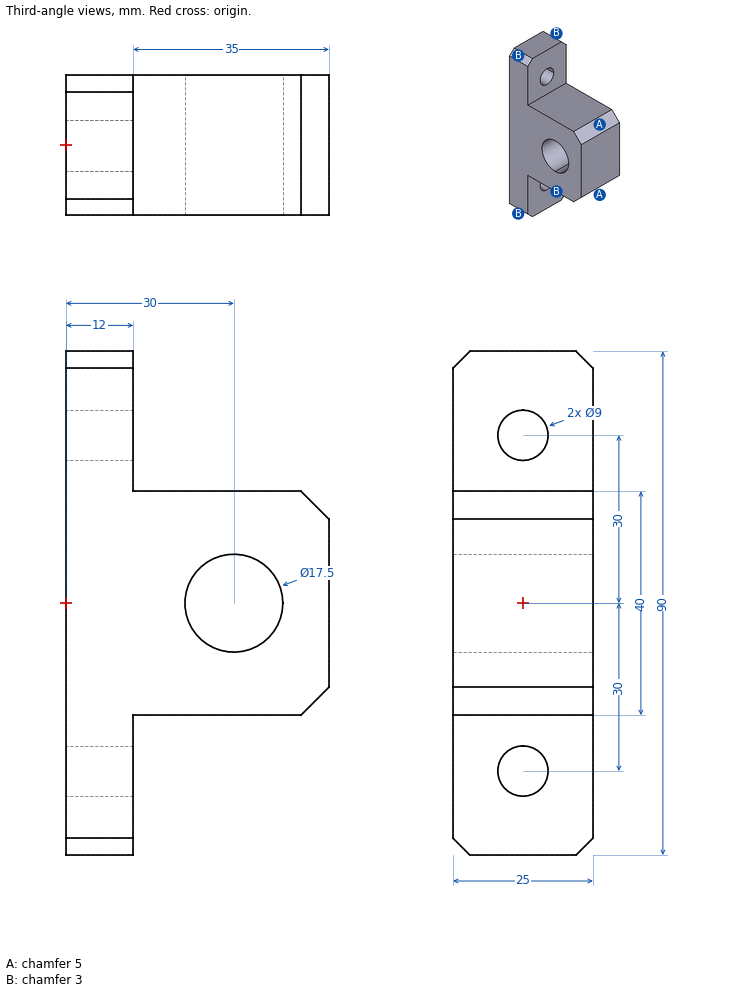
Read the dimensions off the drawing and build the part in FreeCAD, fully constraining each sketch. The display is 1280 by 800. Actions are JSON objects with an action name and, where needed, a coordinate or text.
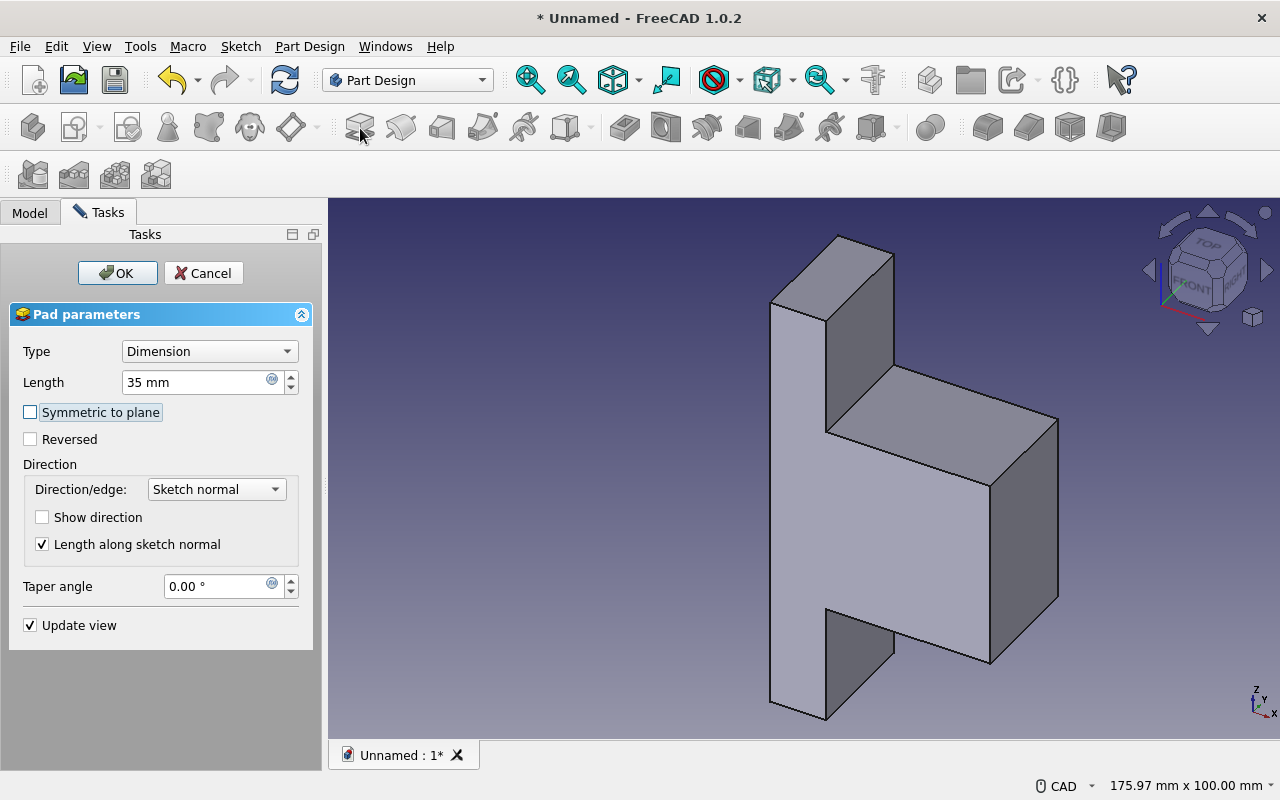
{"action": "left_click", "coordinate": [118, 273]}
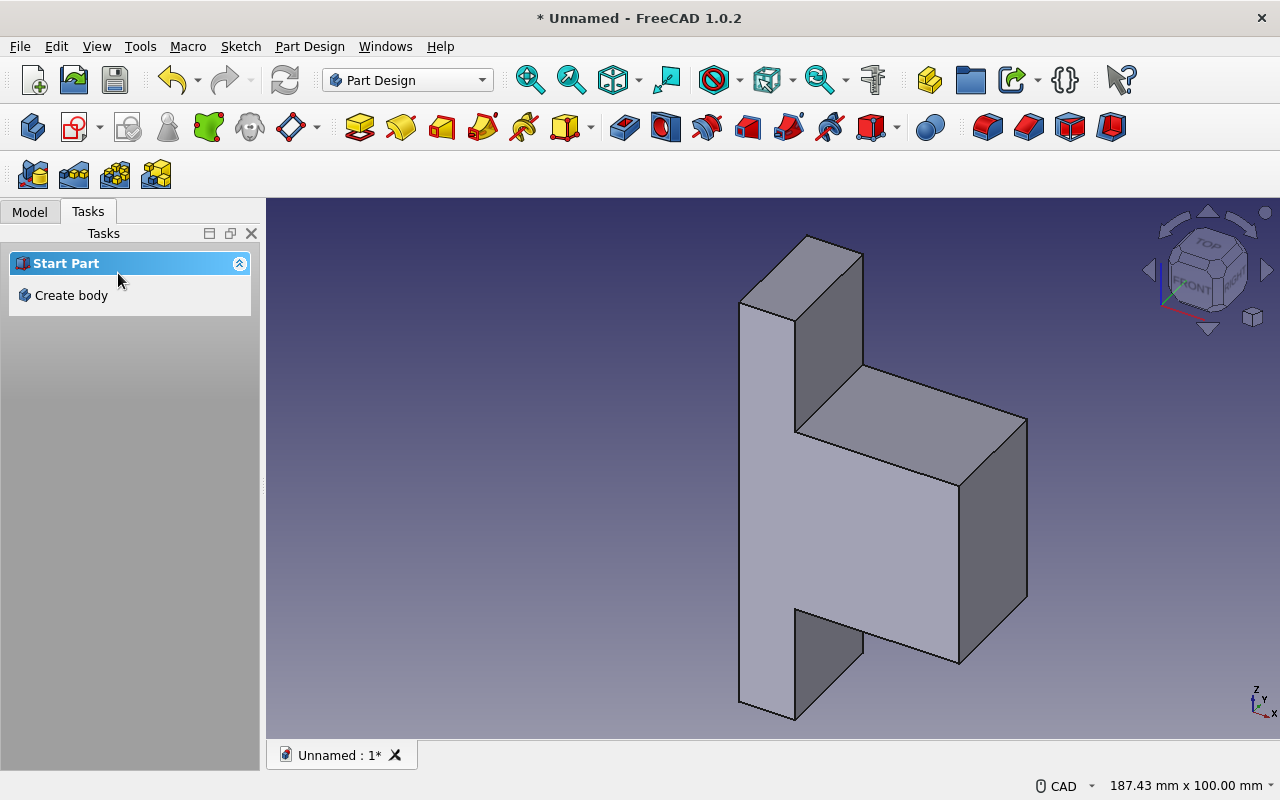
{"action": "left_click", "coordinate": [531, 80]}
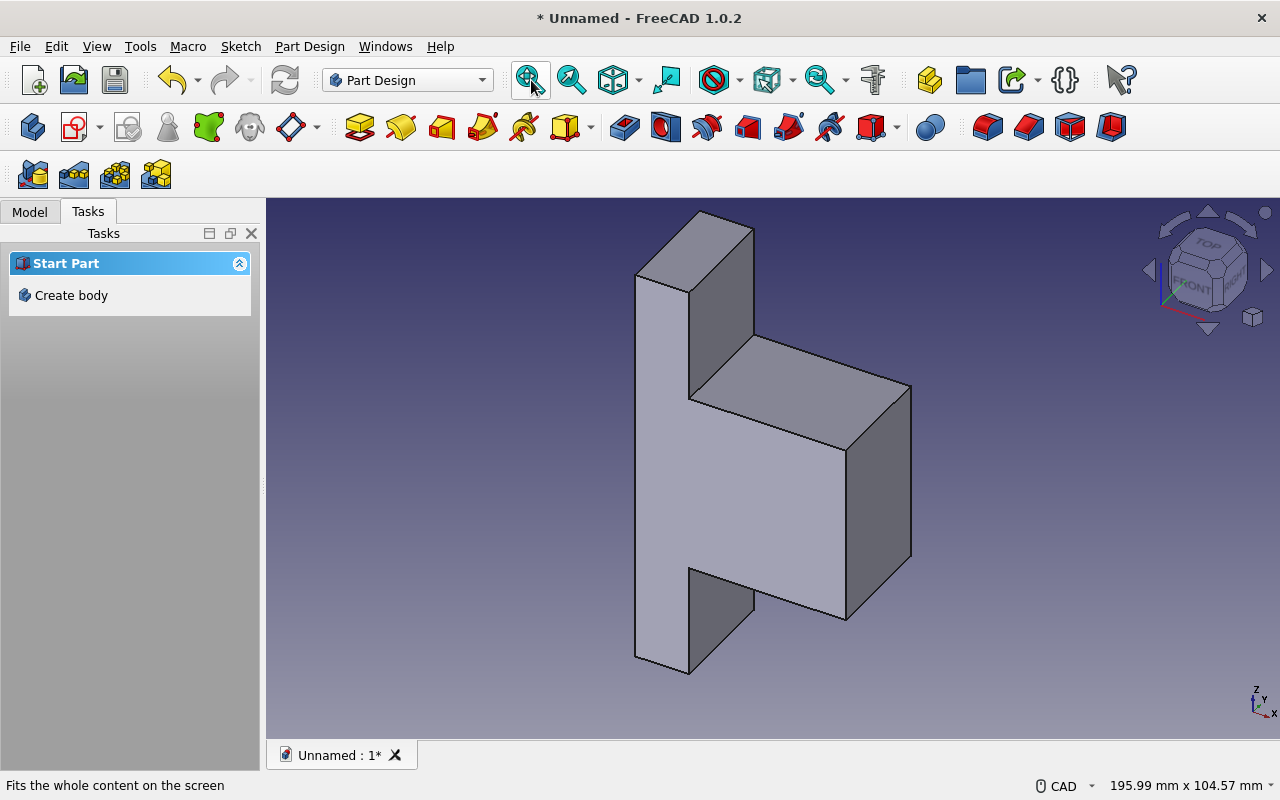
{"action": "left_click", "coordinate": [741, 500]}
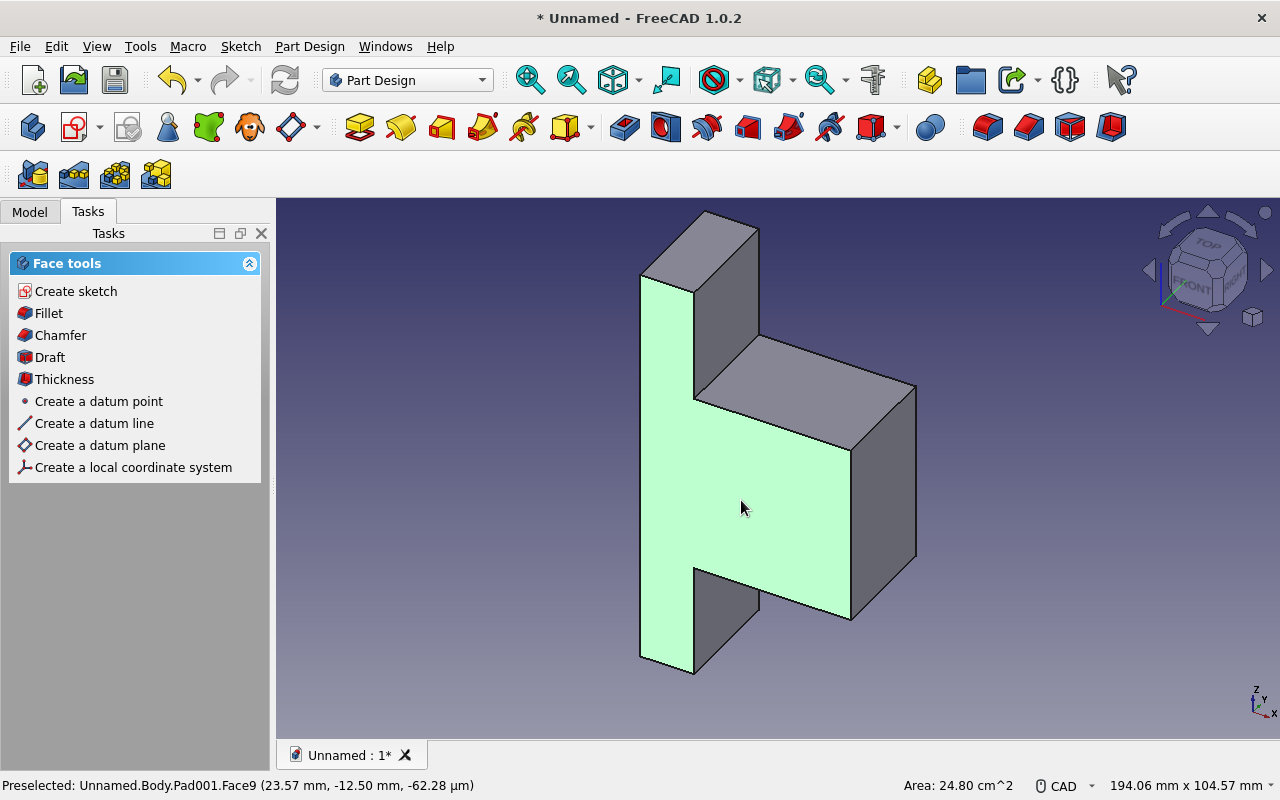
{"action": "left_click", "coordinate": [74, 128]}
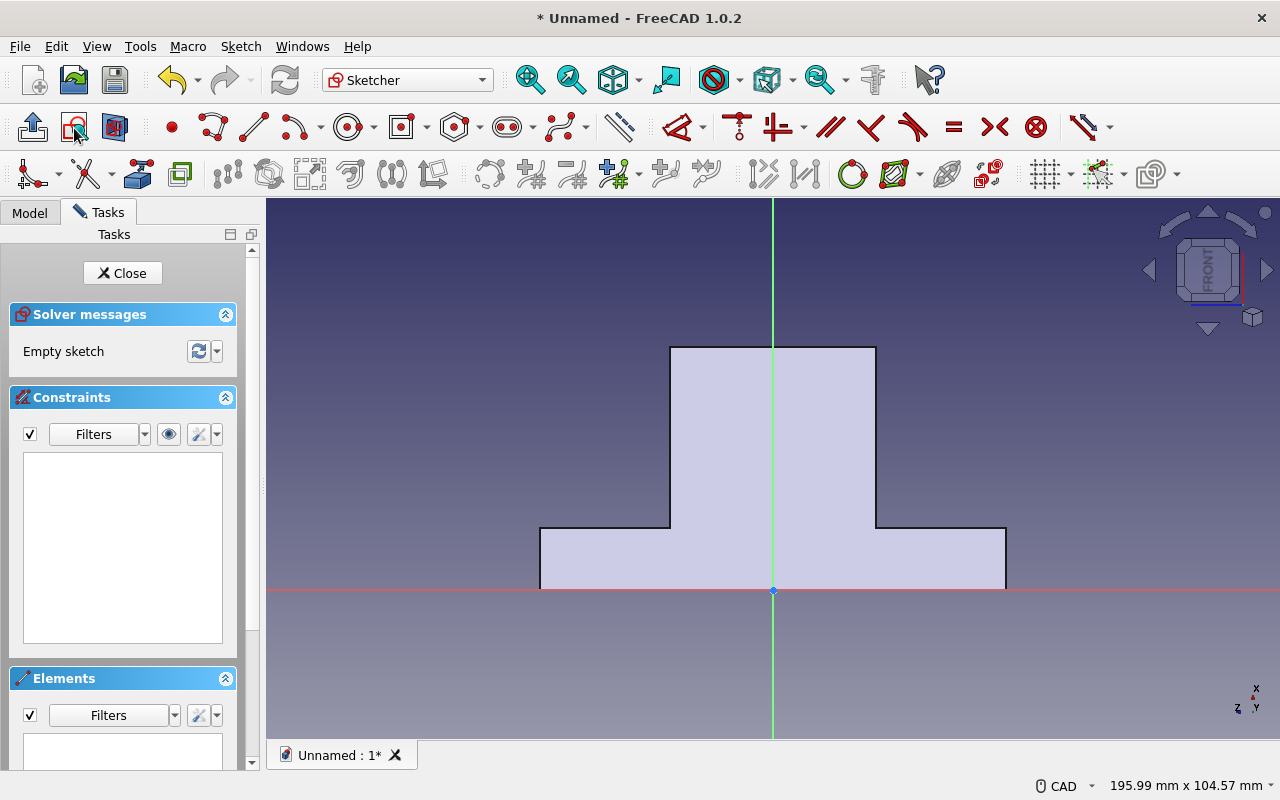
{"action": "scroll", "coordinate": [856, 516], "scroll_direction": "up", "scroll_amount": 3}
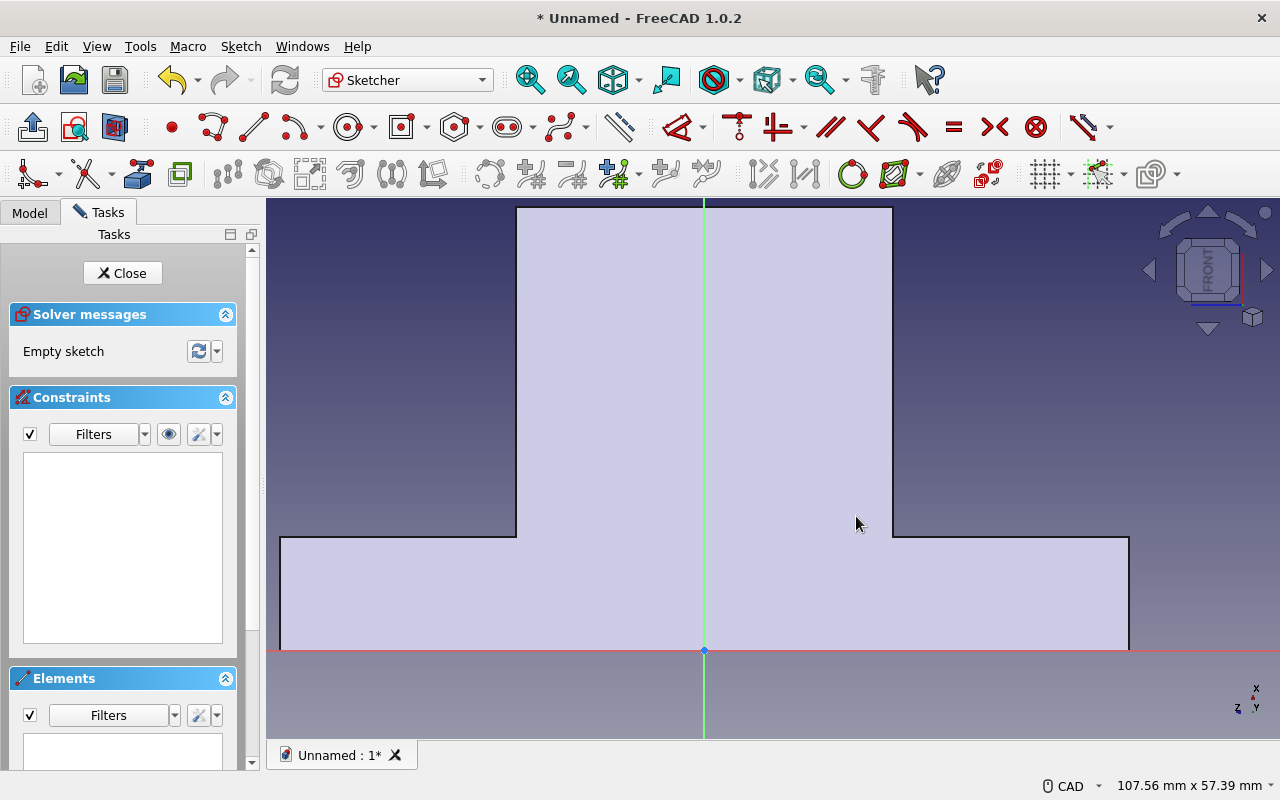
{"action": "left_click", "coordinate": [348, 128]}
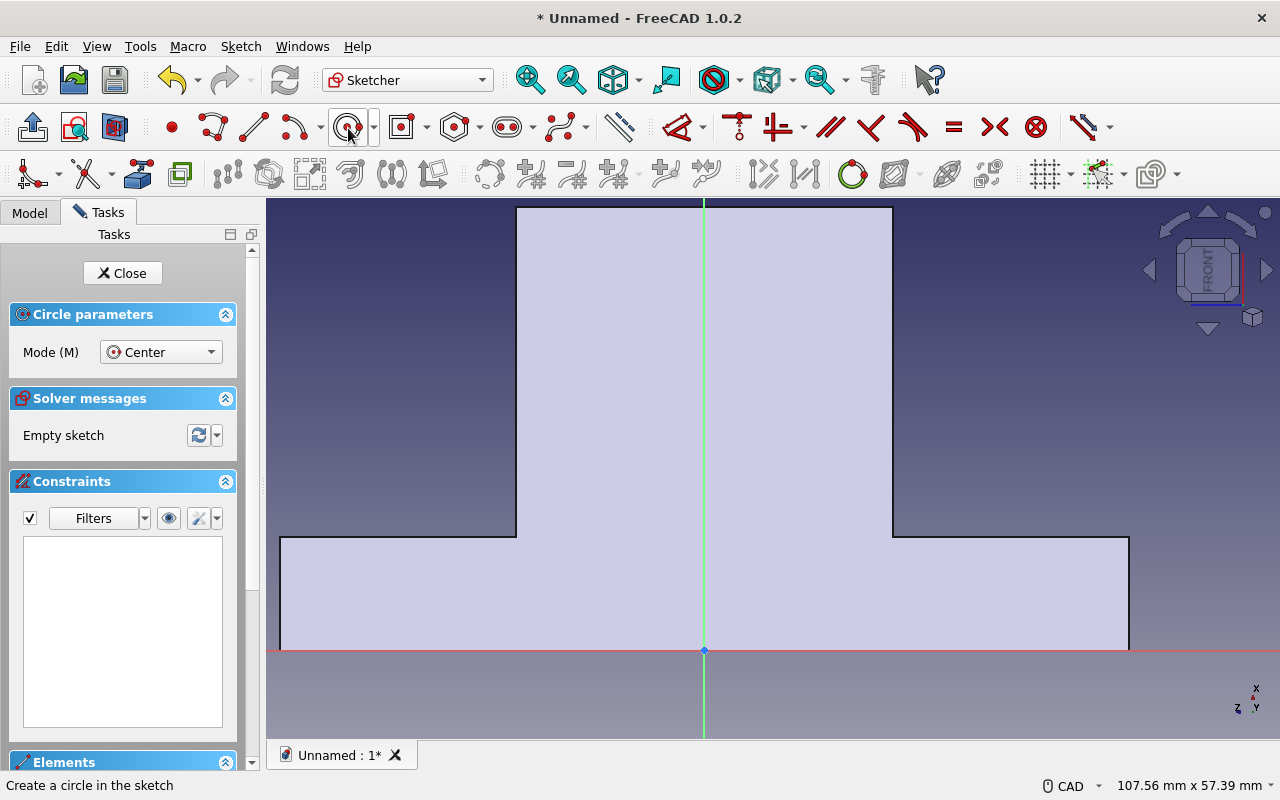
{"action": "left_click", "coordinate": [704, 368]}
{"action": "left_click", "coordinate": [763, 309]}
{"action": "key", "text": "Escape"}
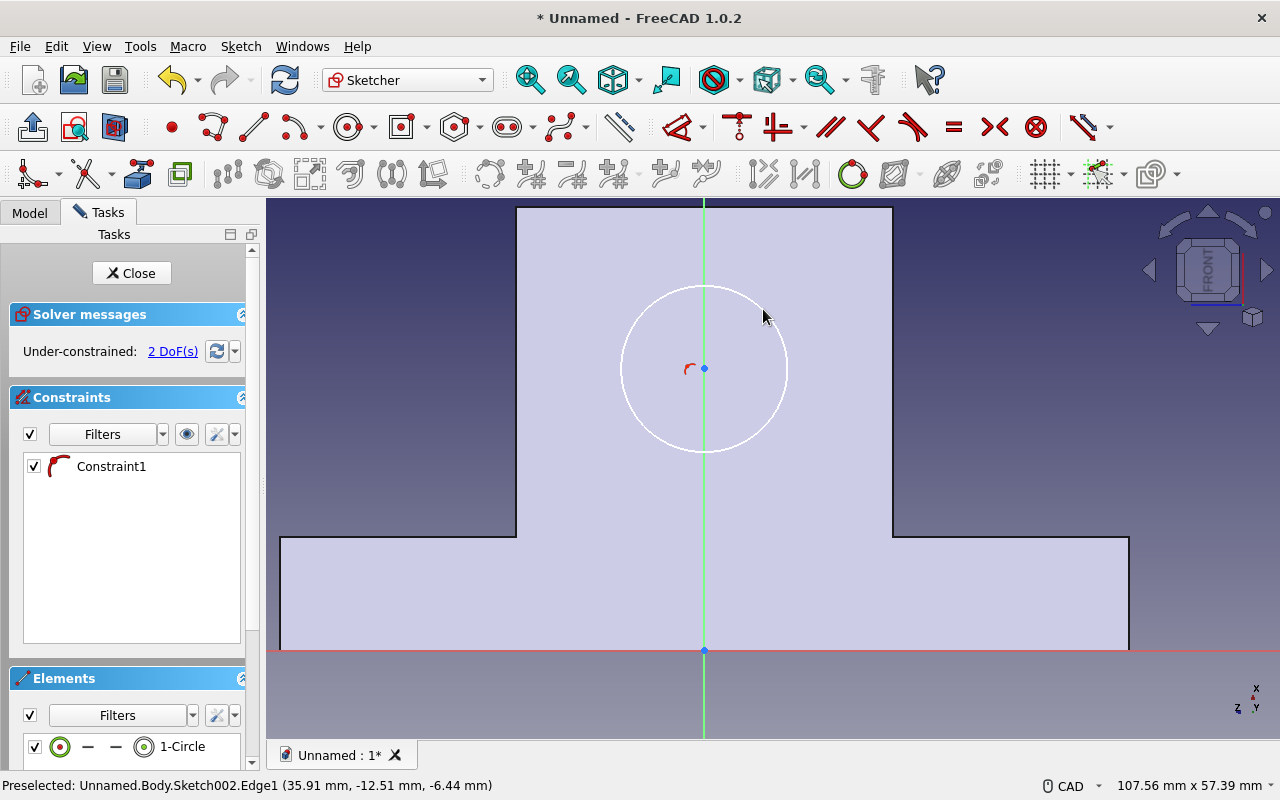
{"action": "left_click", "coordinate": [676, 128]}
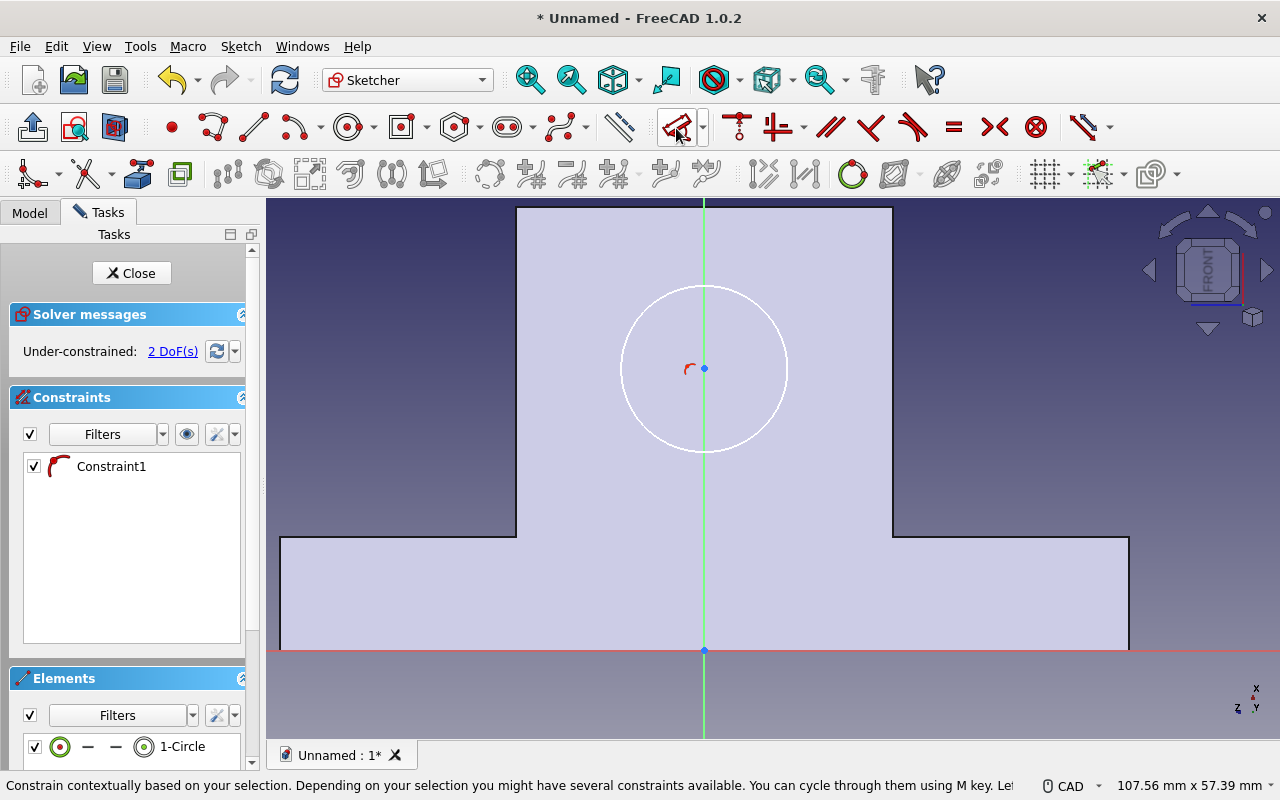
{"action": "left_click", "coordinate": [763, 310]}
{"action": "left_click", "coordinate": [786, 287]}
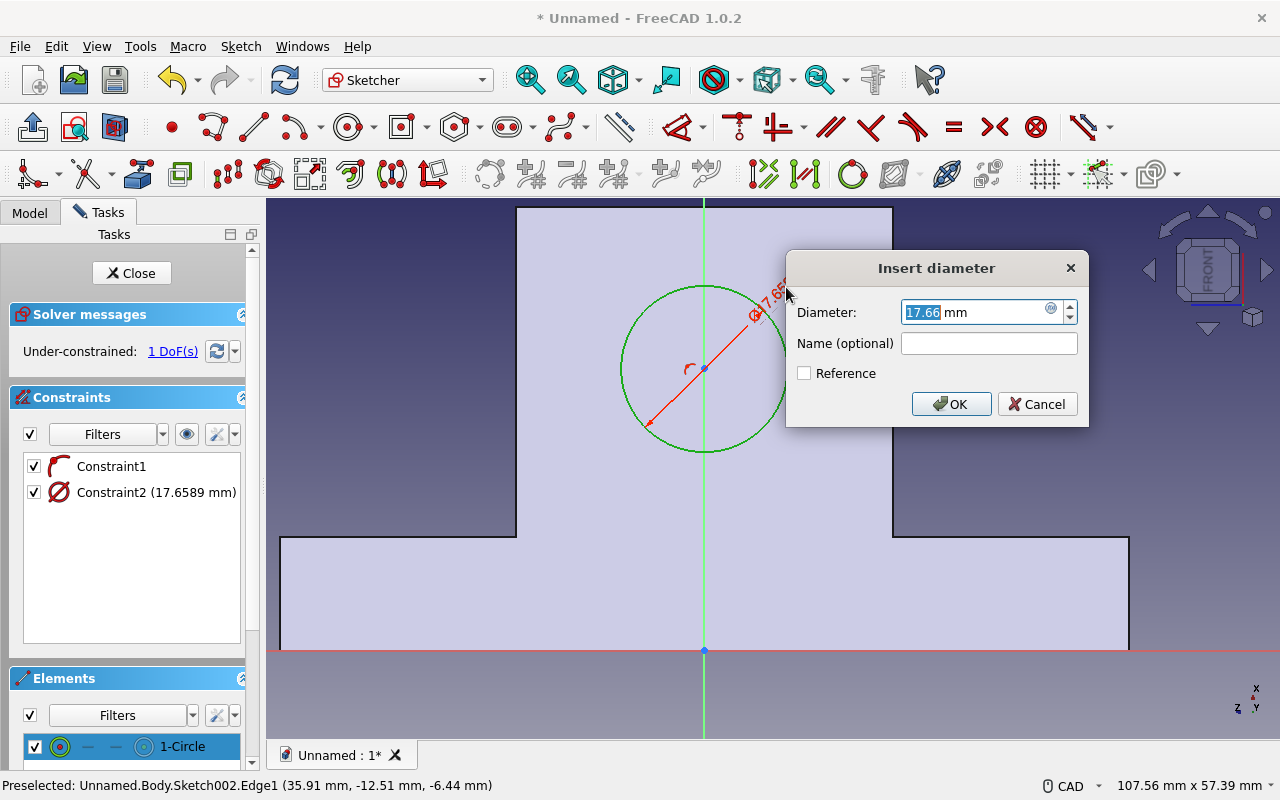
{"action": "type", "text": "17.5"}
{"action": "key", "text": "Return"}